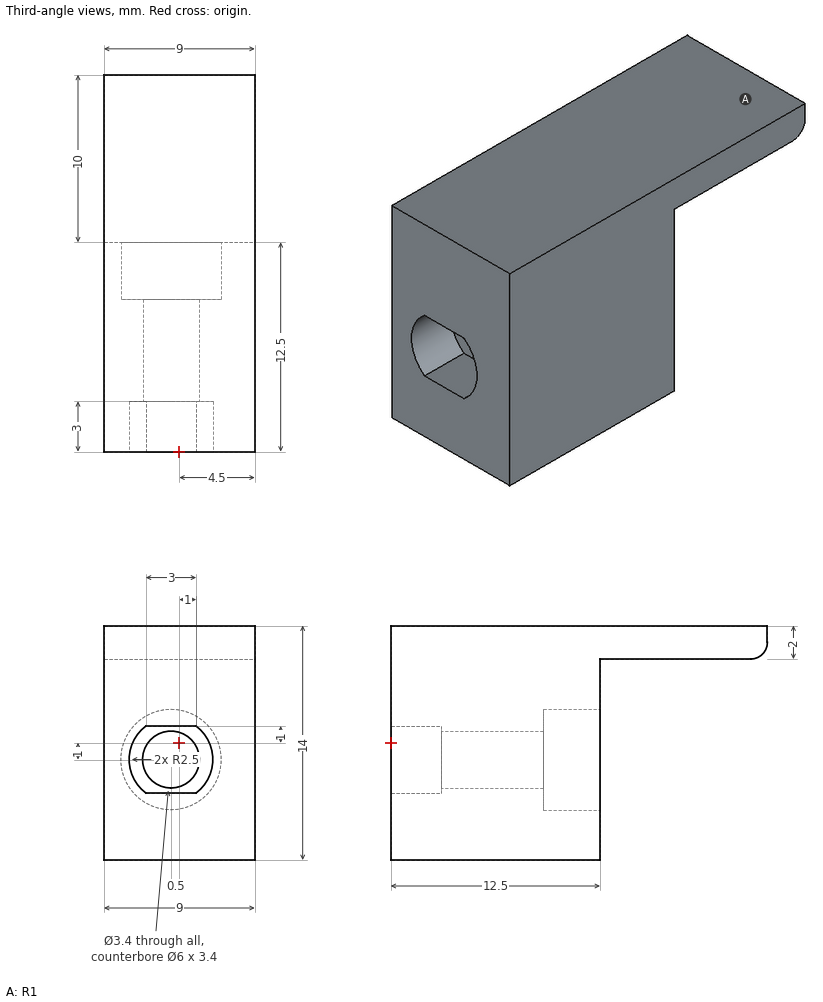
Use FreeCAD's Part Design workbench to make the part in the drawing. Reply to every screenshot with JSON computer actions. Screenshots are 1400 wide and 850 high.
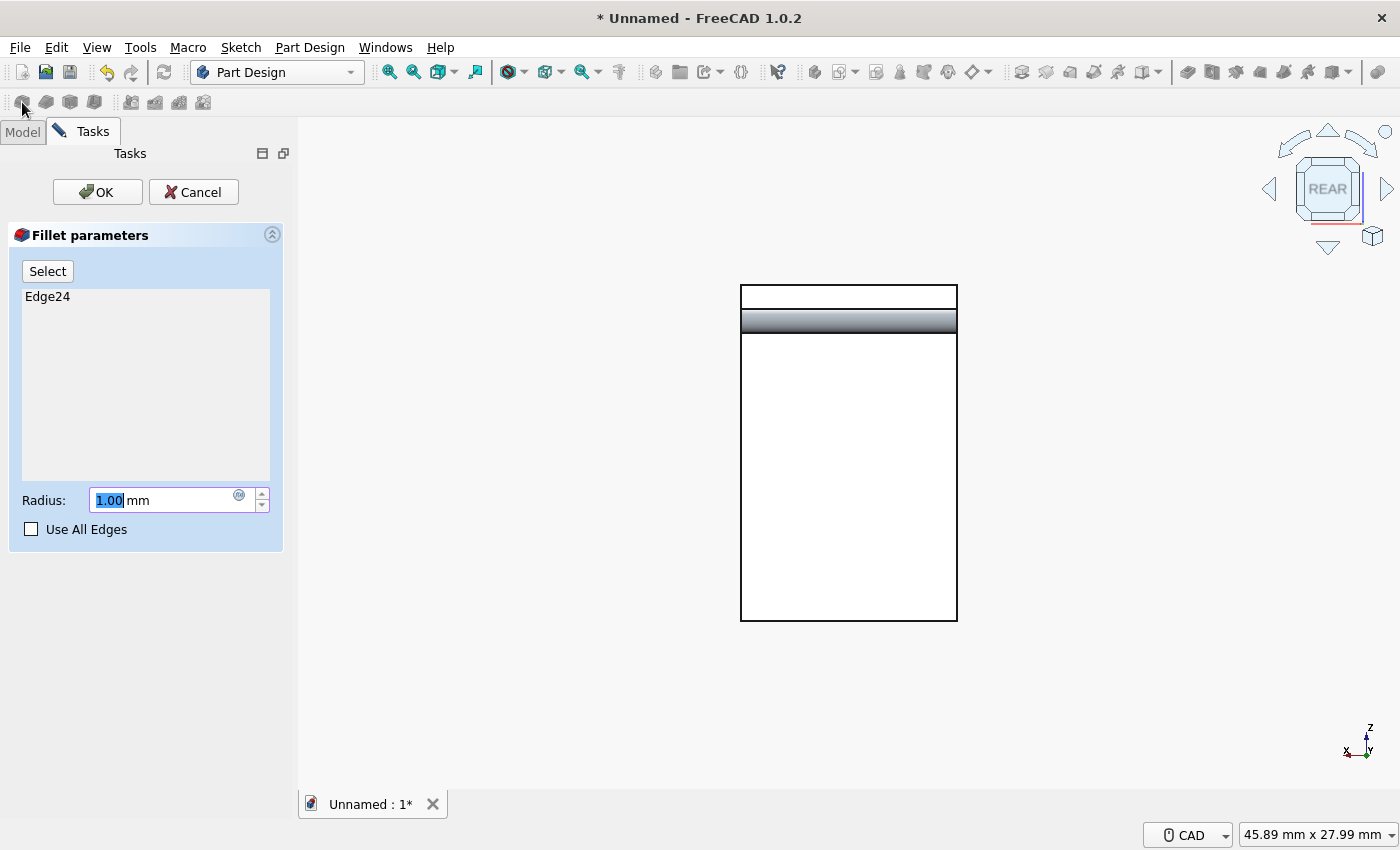
{"action": "type", "text": "1"}
{"action": "key", "text": "Tab"}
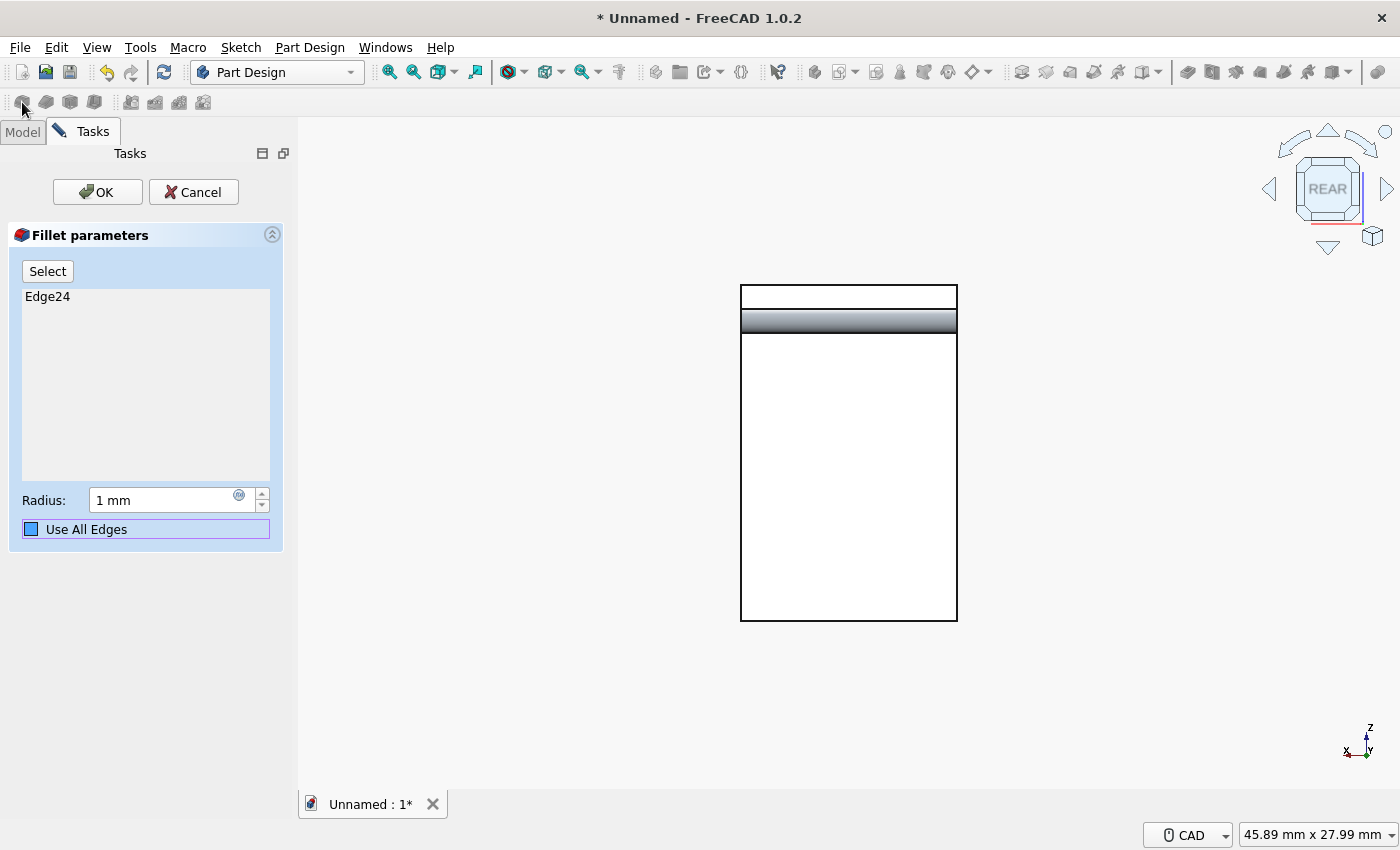
{"action": "left_click", "coordinate": [98, 192]}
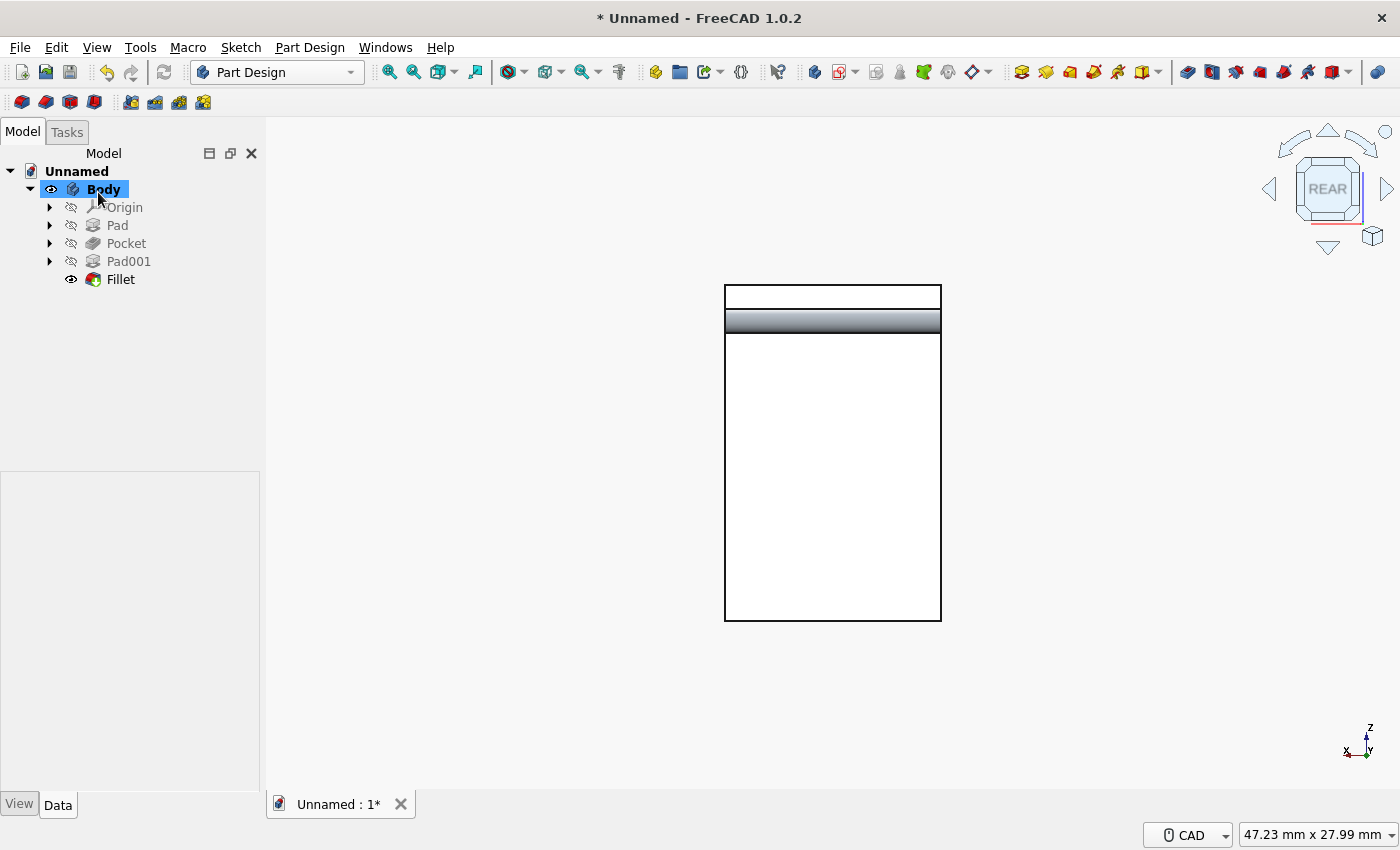
{"action": "left_click", "coordinate": [833, 476]}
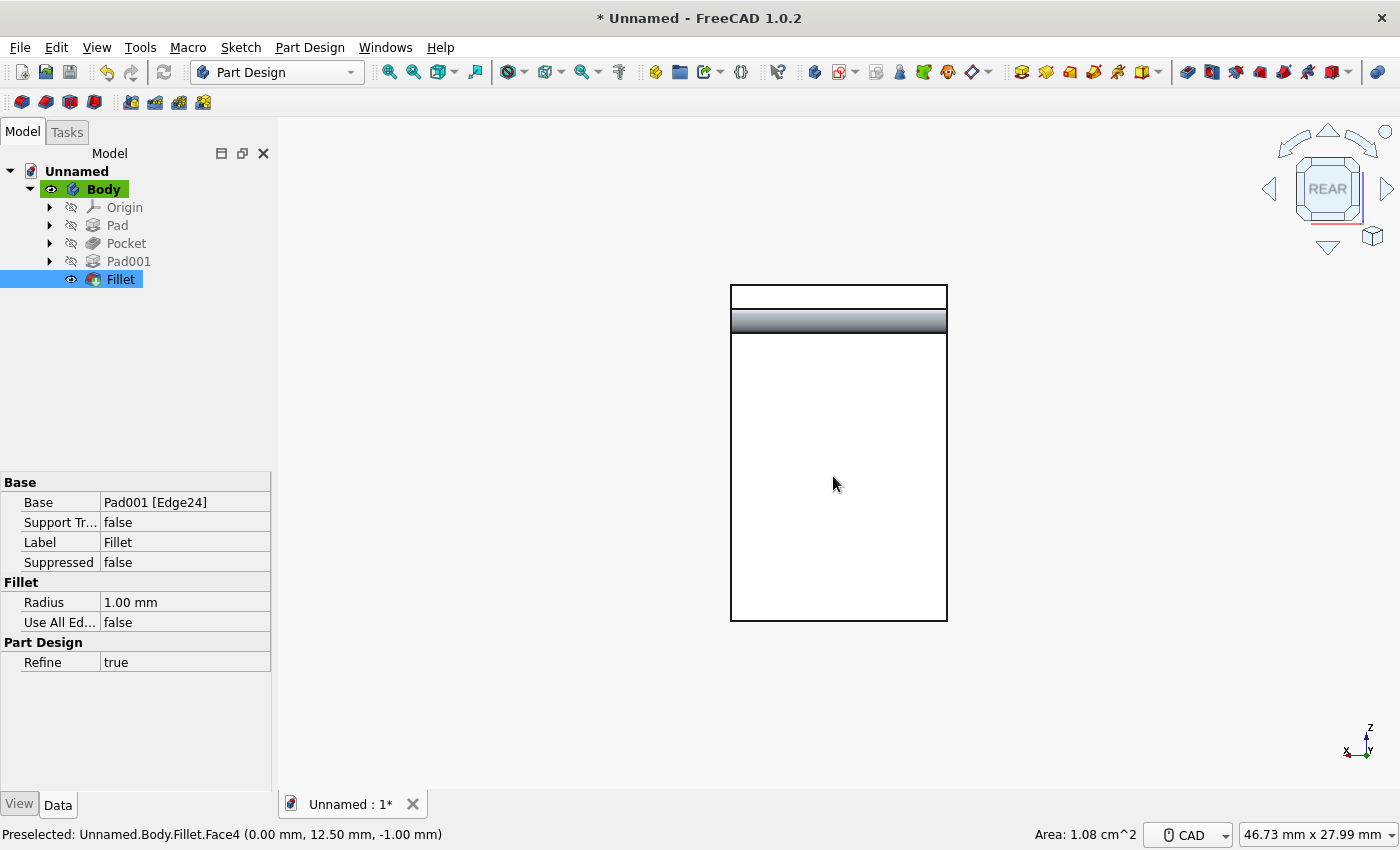
{"action": "left_click", "coordinate": [840, 72]}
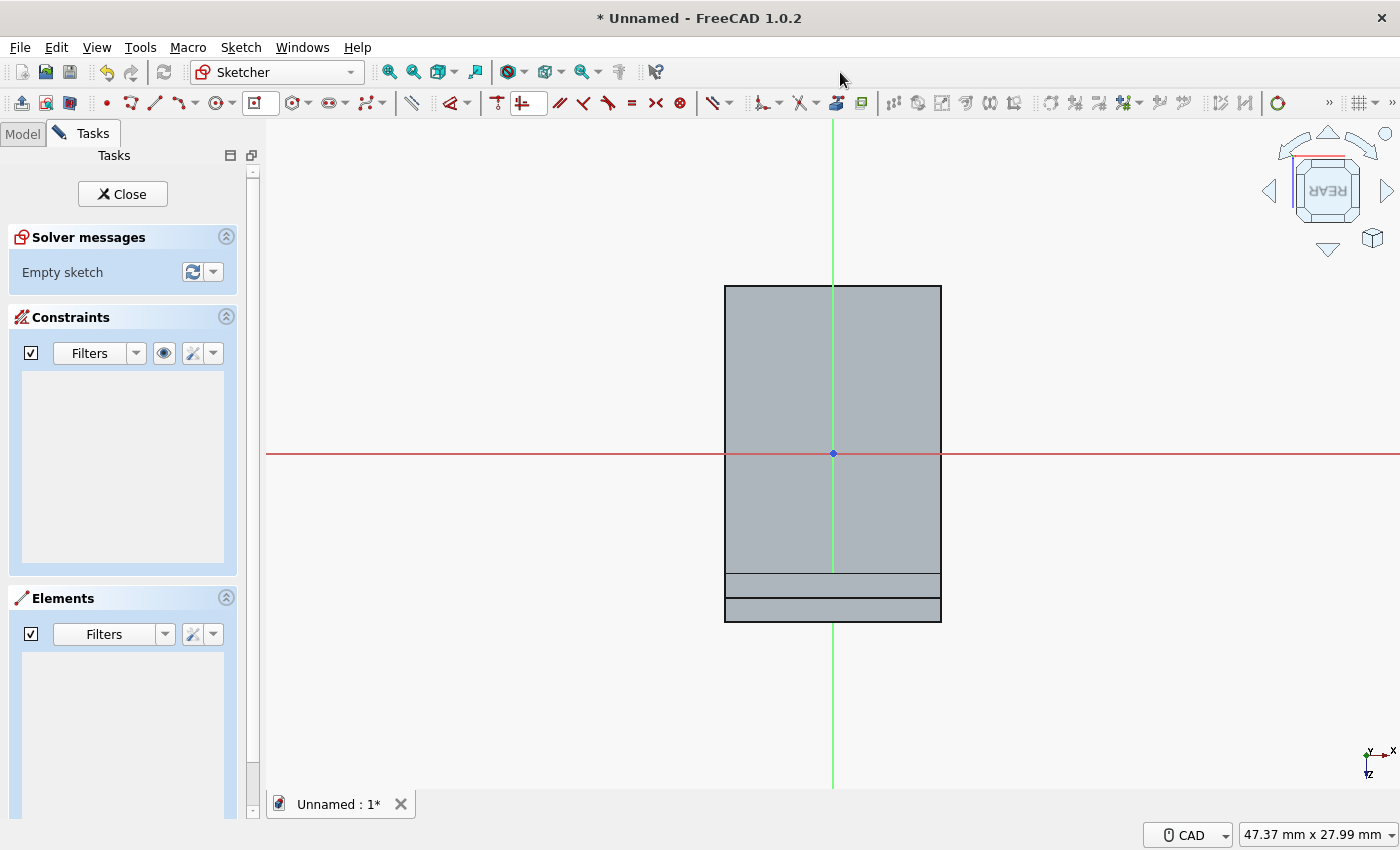
{"action": "scroll", "coordinate": [835, 424], "scroll_direction": "up", "scroll_amount": 8}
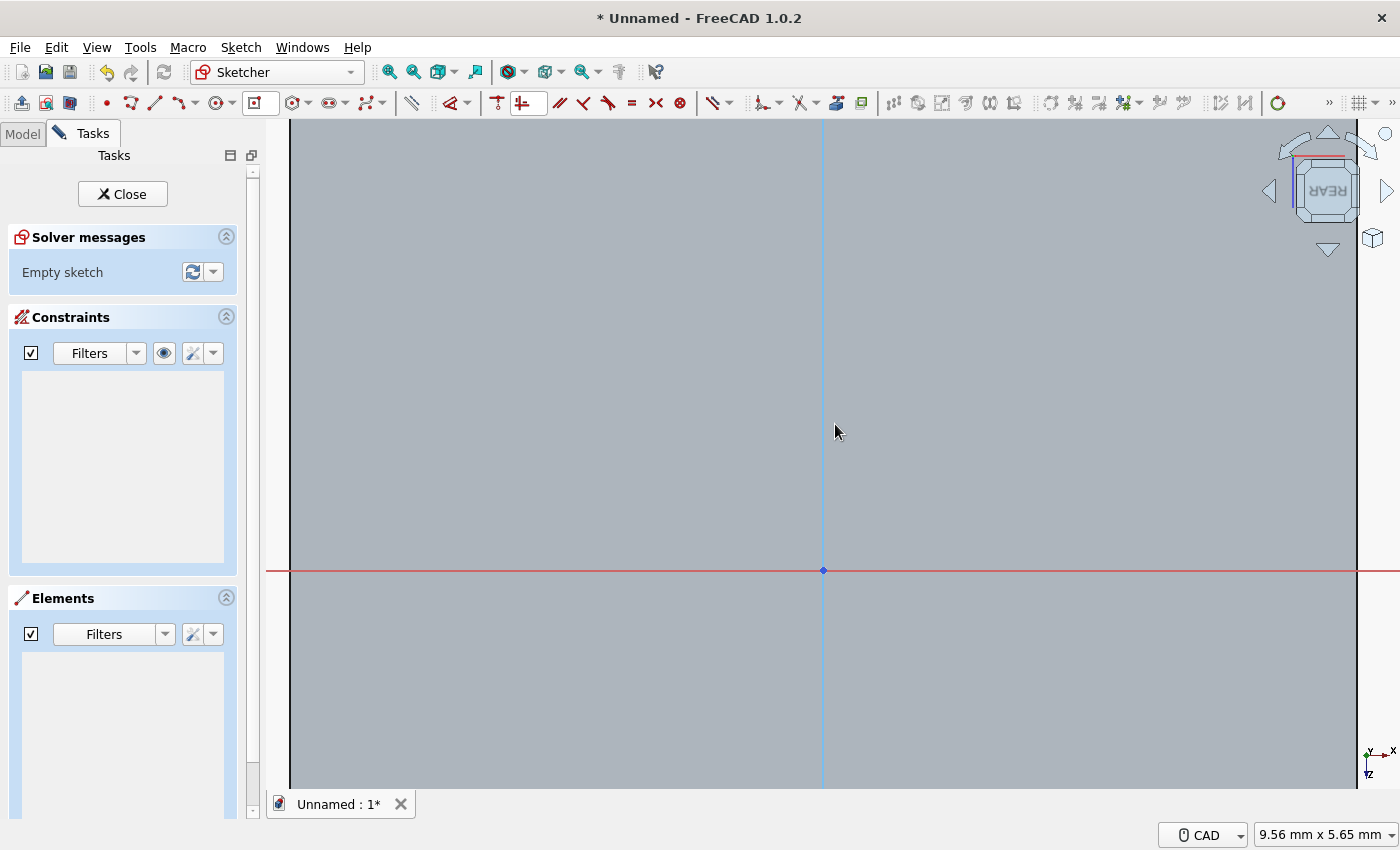
{"action": "left_click", "coordinate": [216, 104]}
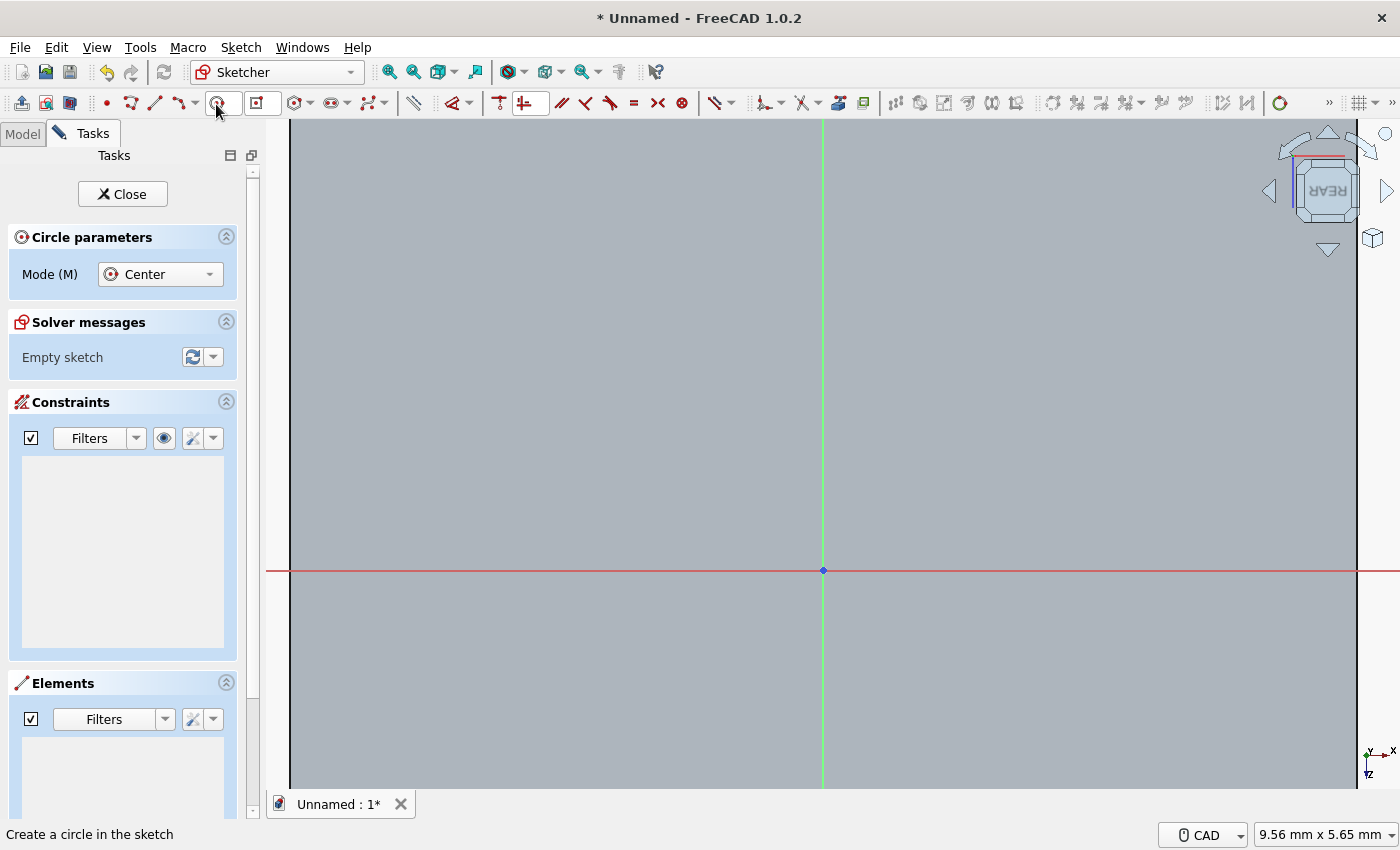
{"action": "left_click", "coordinate": [764, 452]}
{"action": "mouse_move", "coordinate": [906, 310]}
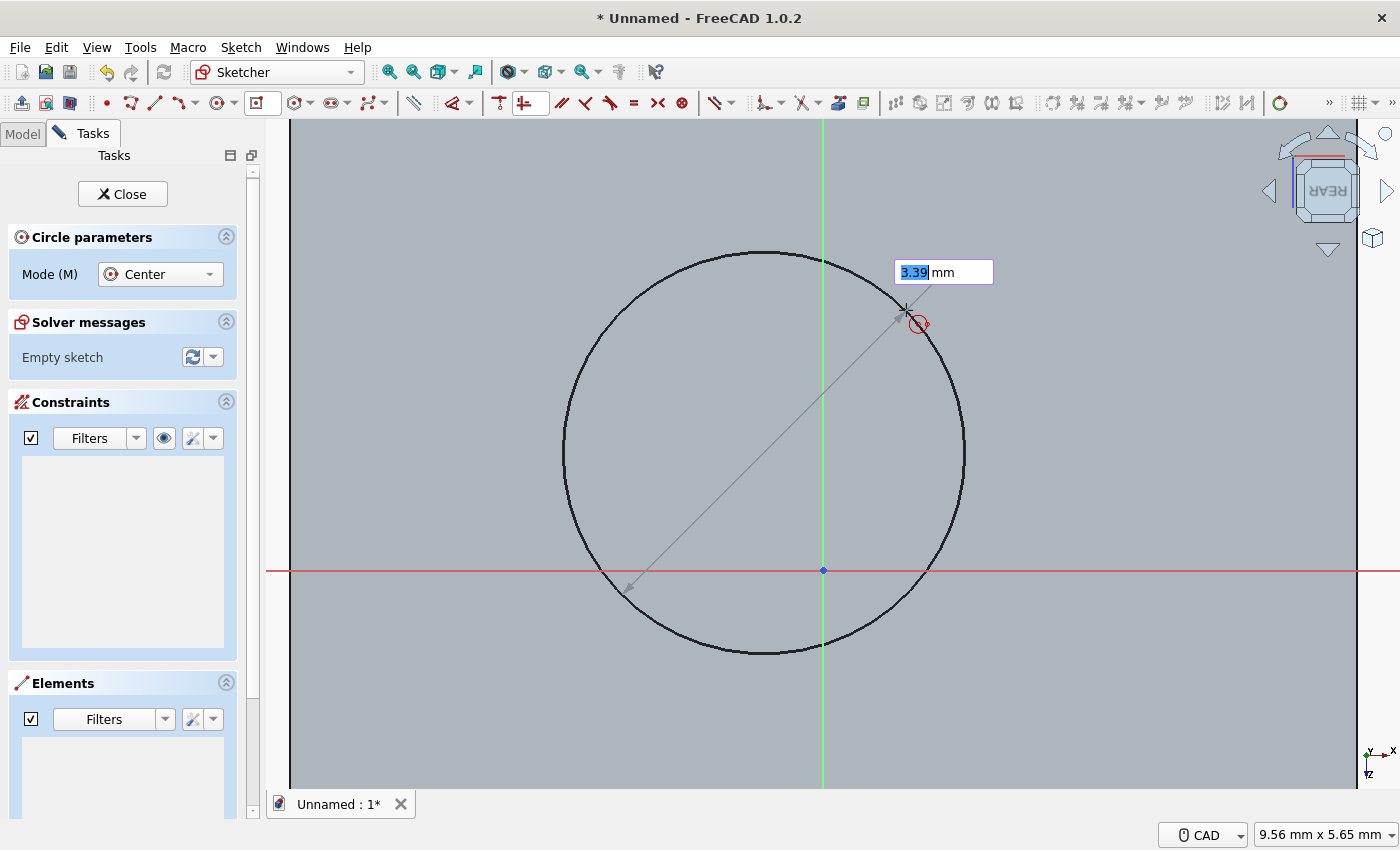
{"action": "type", "text": "3.4"}
{"action": "key", "text": "Return"}
{"action": "key", "text": "Escape"}